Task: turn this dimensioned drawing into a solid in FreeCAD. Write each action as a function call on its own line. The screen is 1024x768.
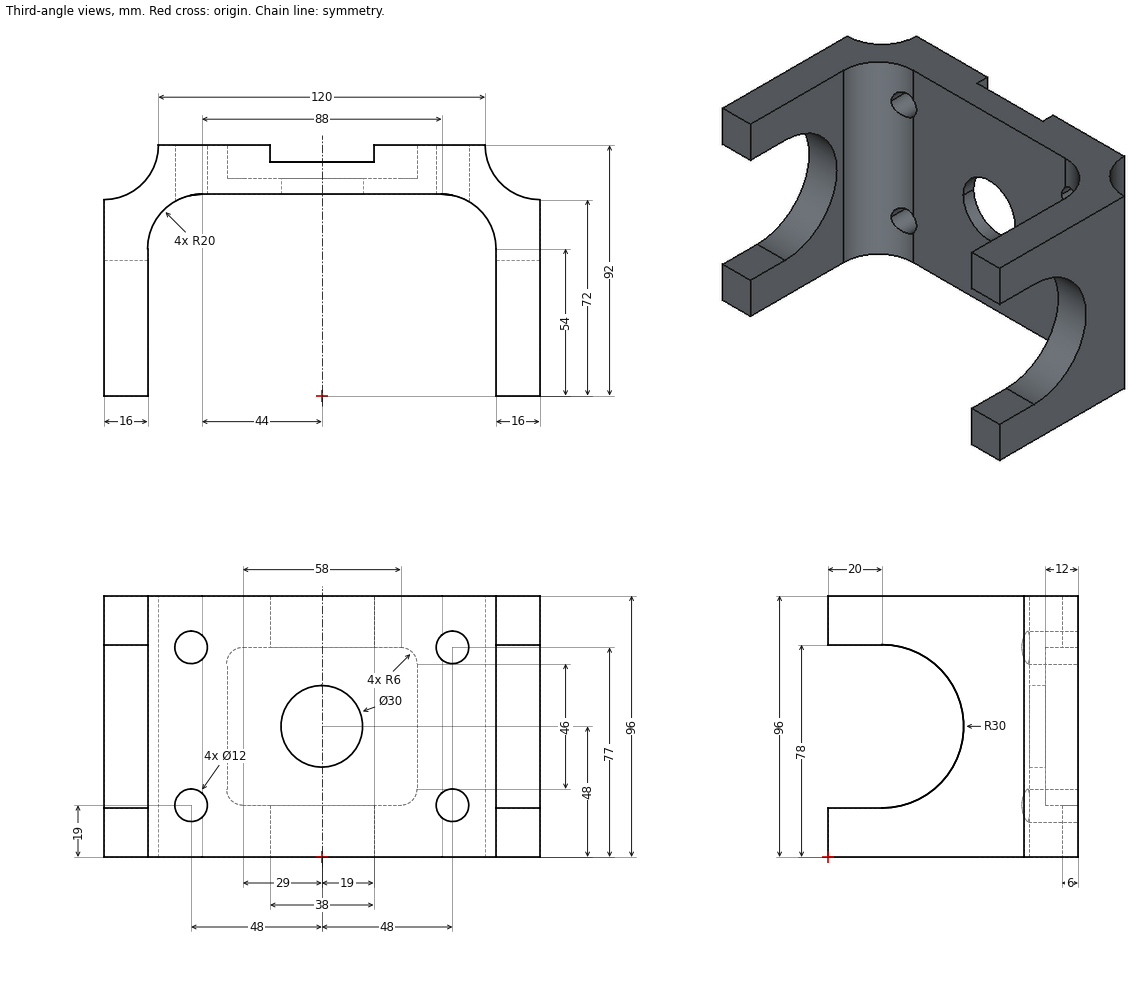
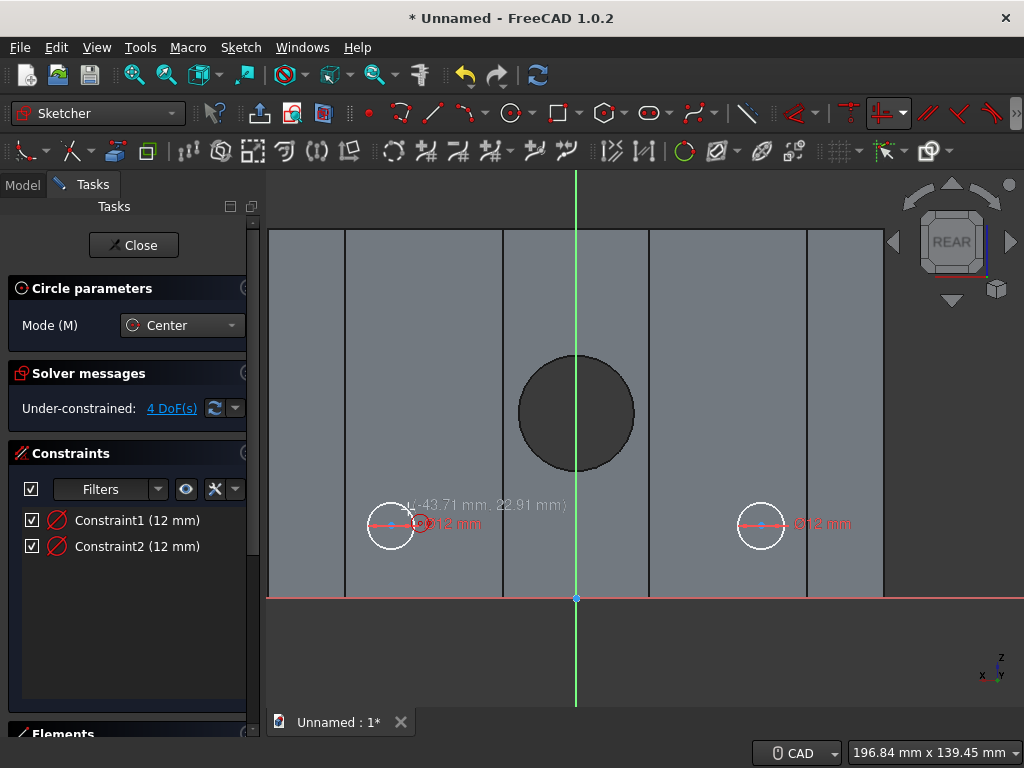
click(391, 302)
move(408, 285)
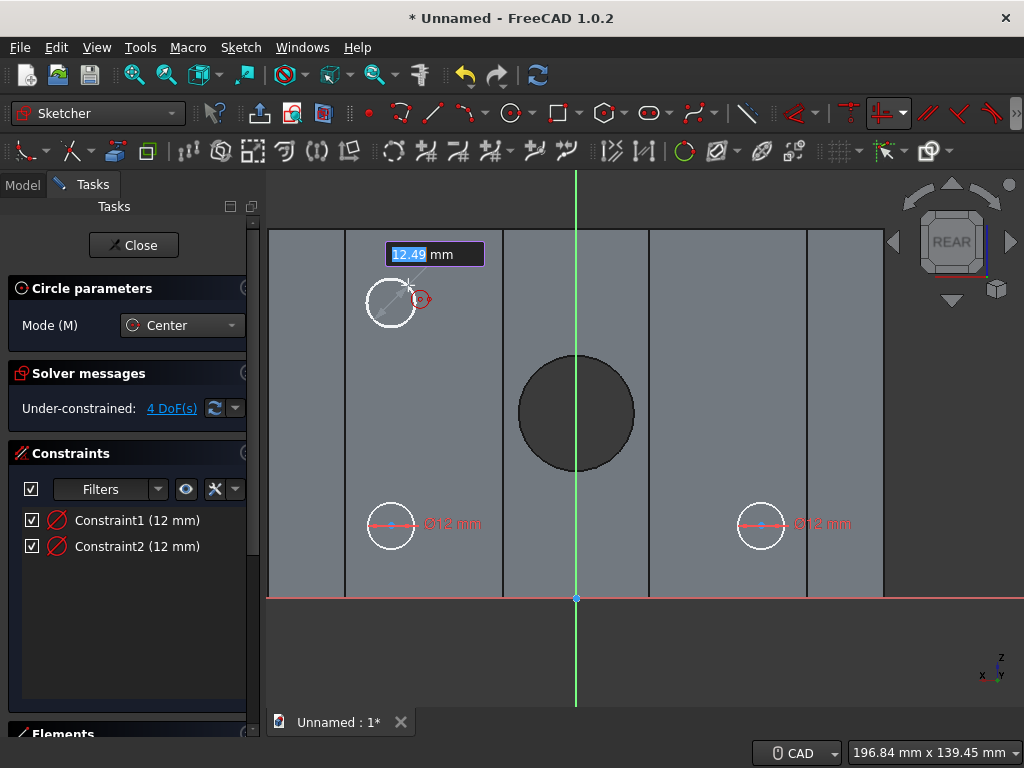
text(12)
key(Return)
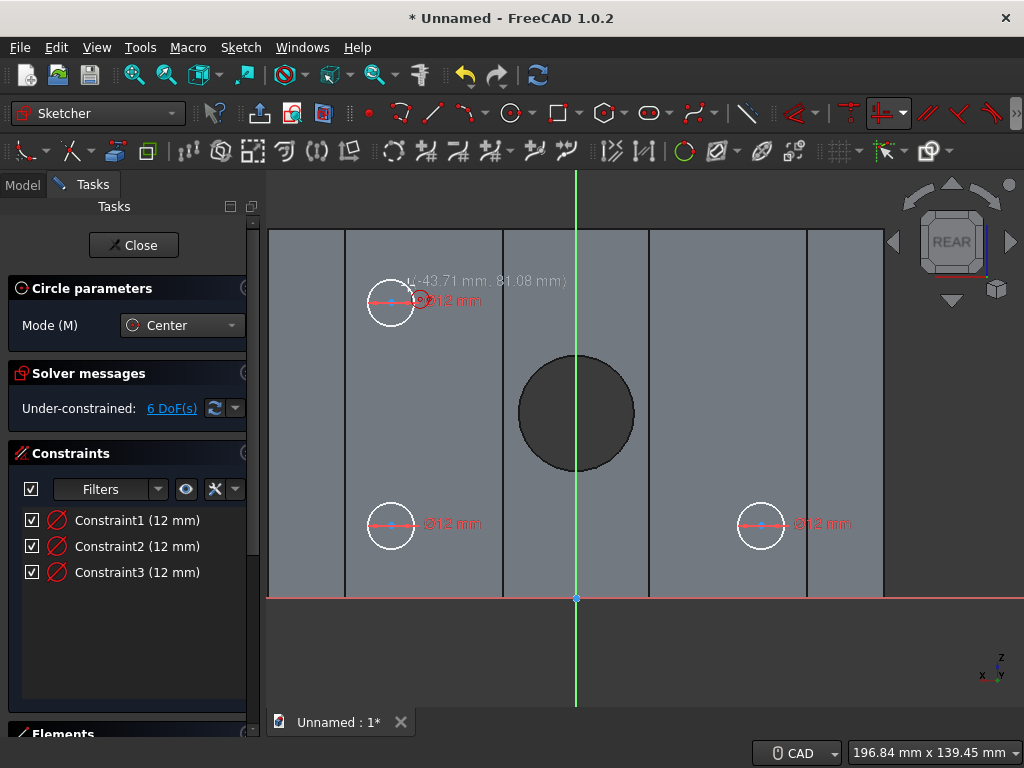
click(761, 302)
move(777, 285)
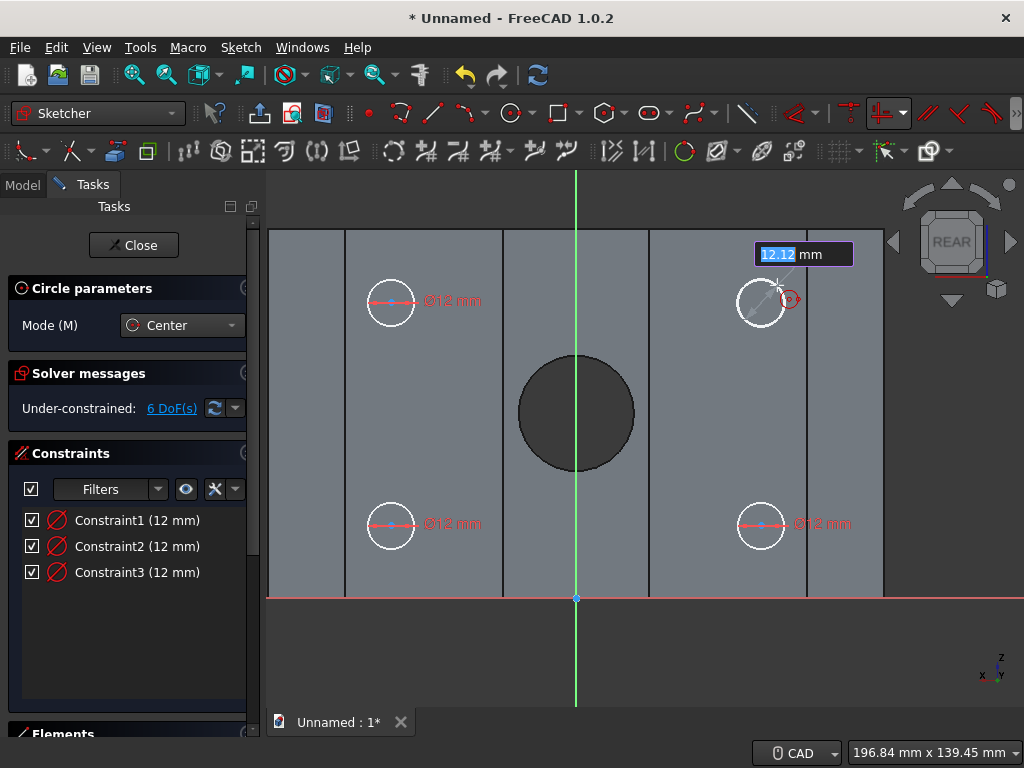
text(12)
key(Return)
key(Escape)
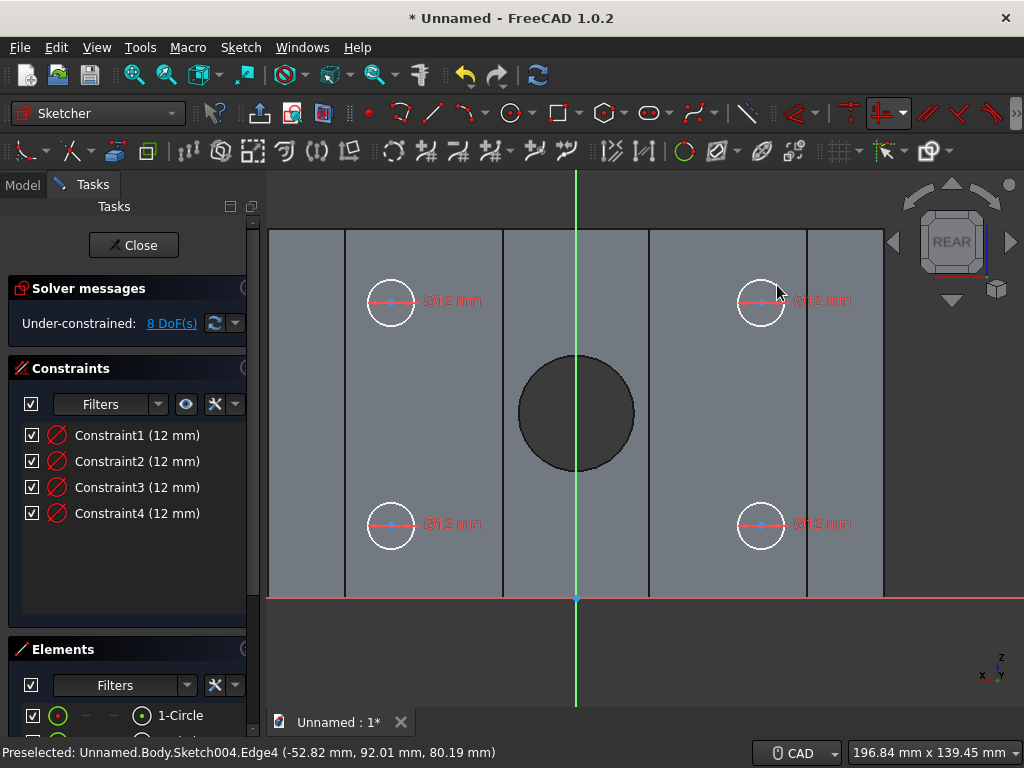
click(761, 526)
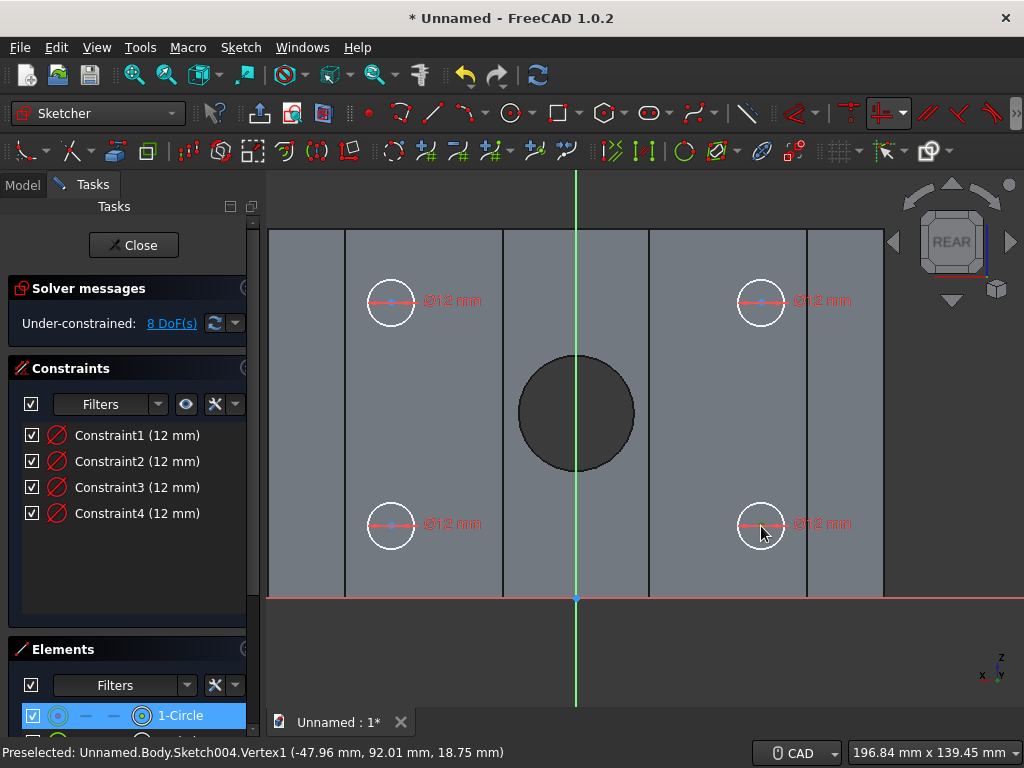
click(391, 526)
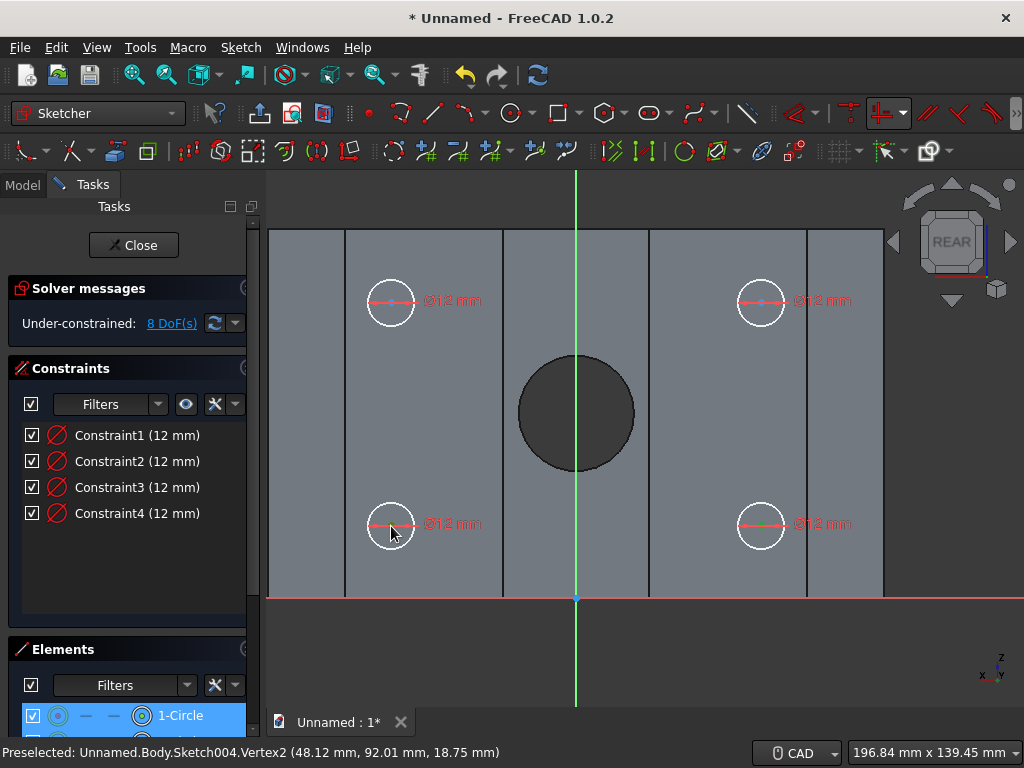
click(576, 645)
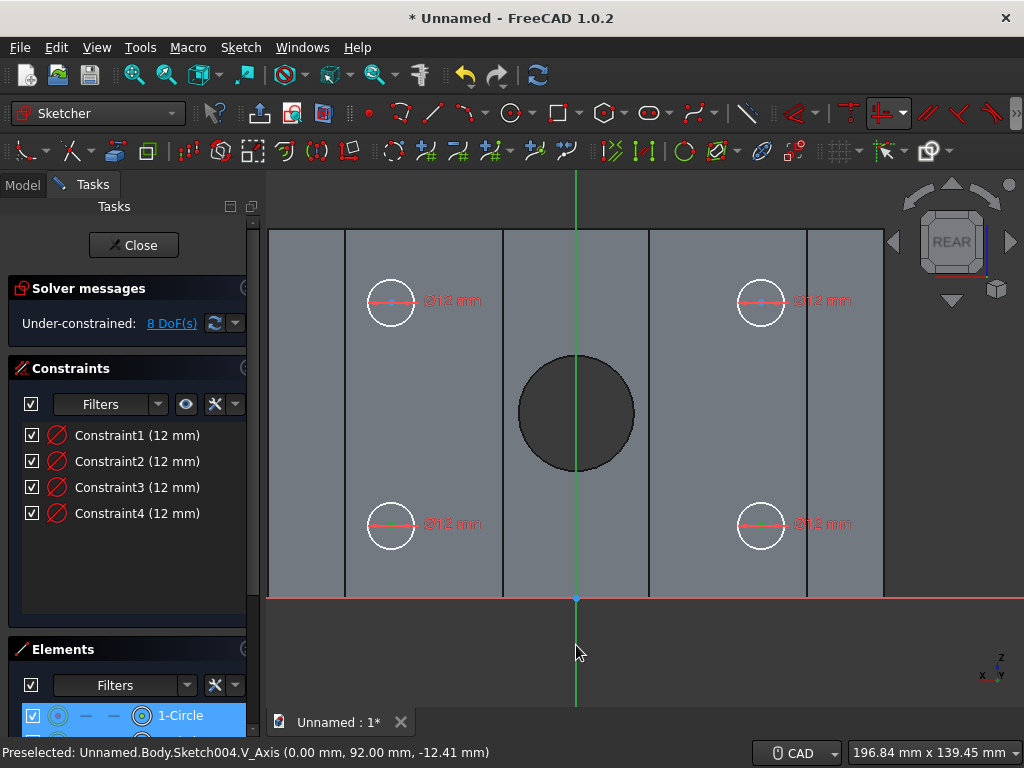
key(s)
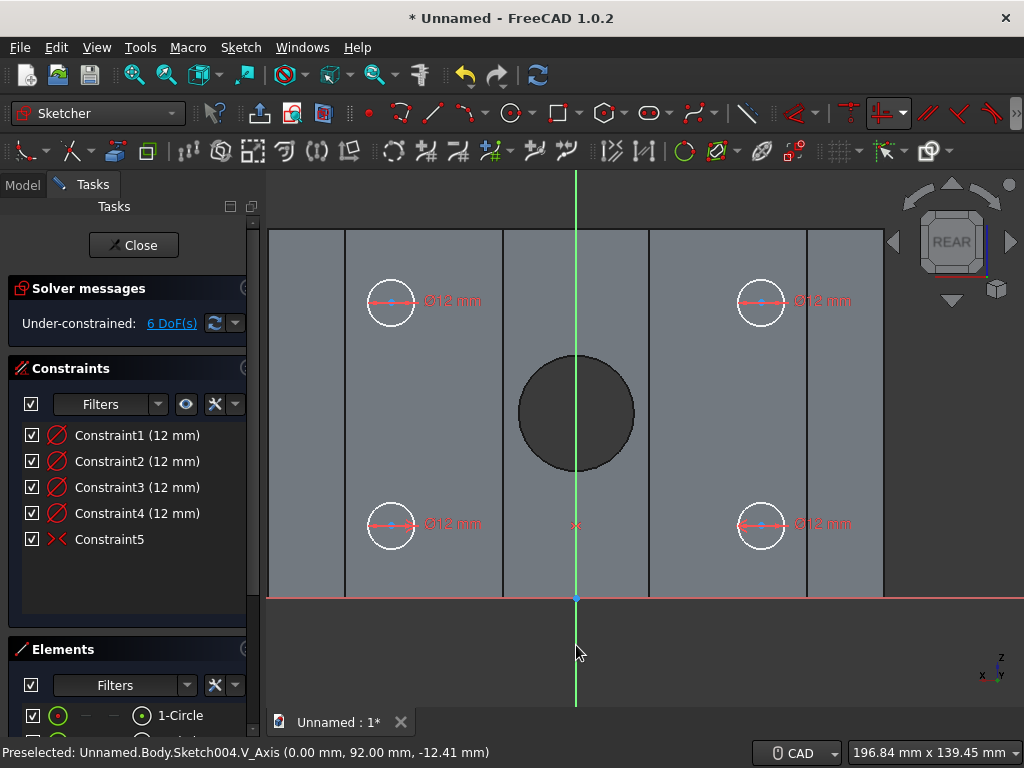
click(391, 303)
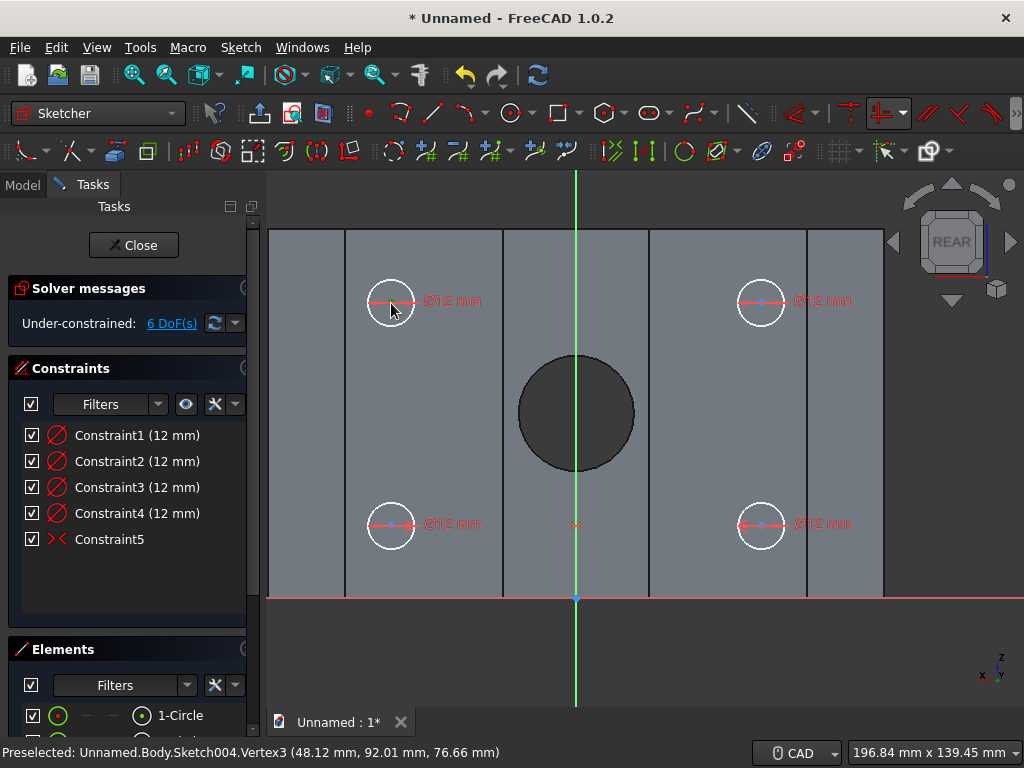
click(761, 303)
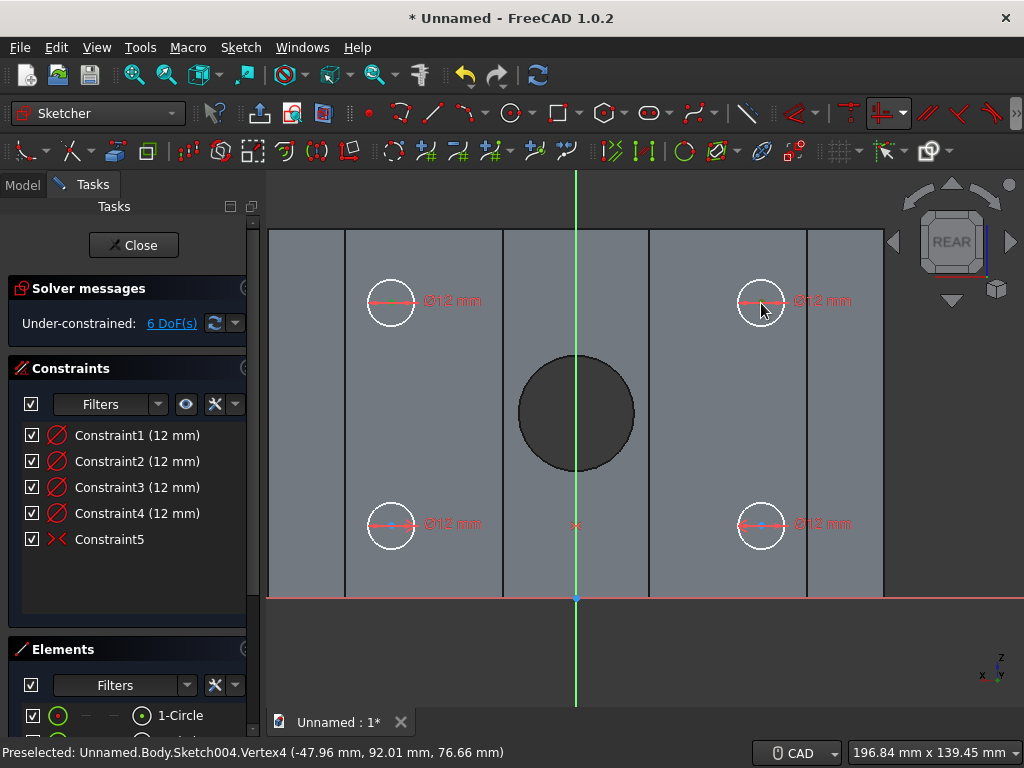
click(576, 645)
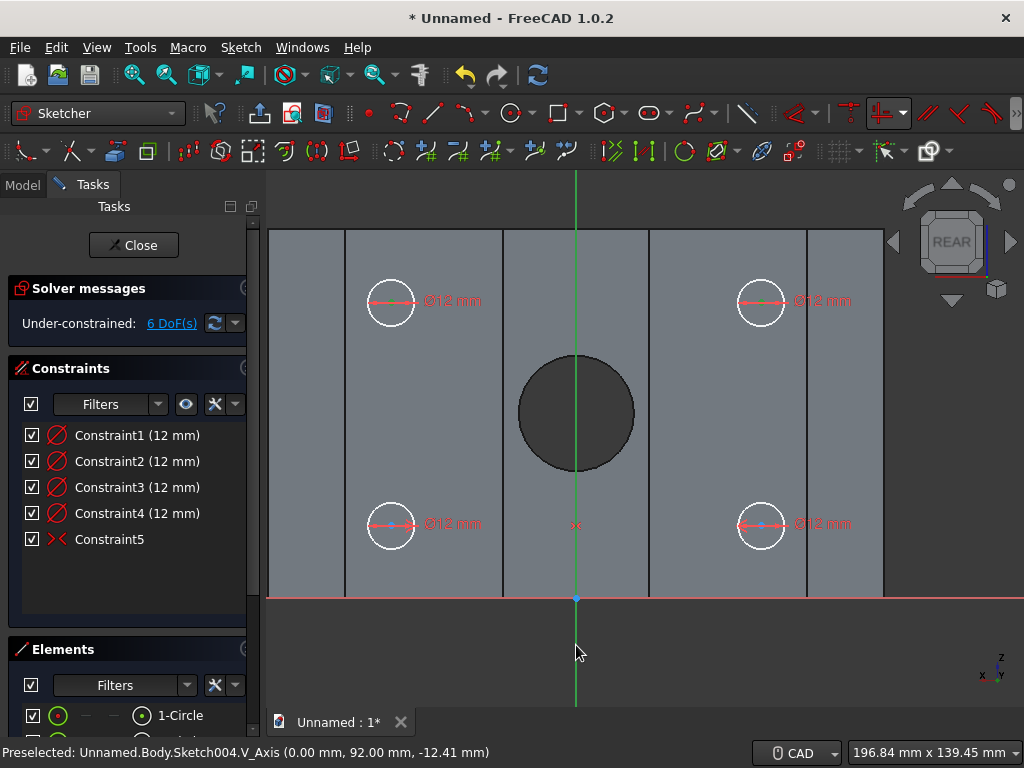
key(s)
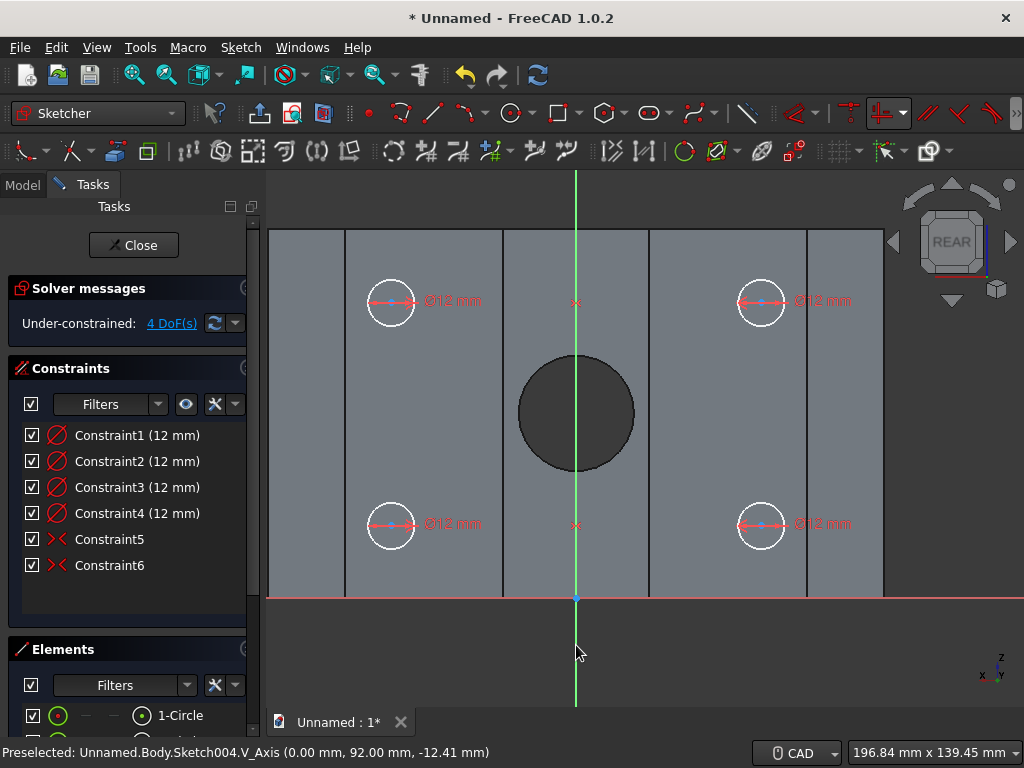
click(794, 114)